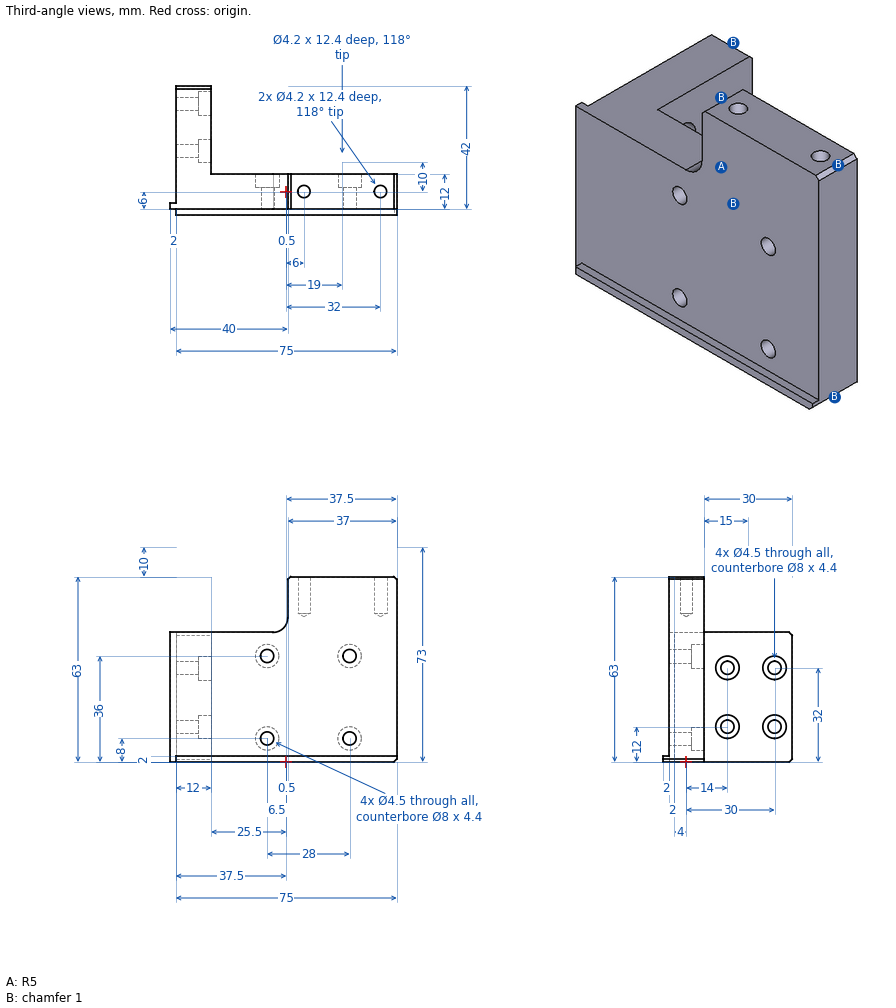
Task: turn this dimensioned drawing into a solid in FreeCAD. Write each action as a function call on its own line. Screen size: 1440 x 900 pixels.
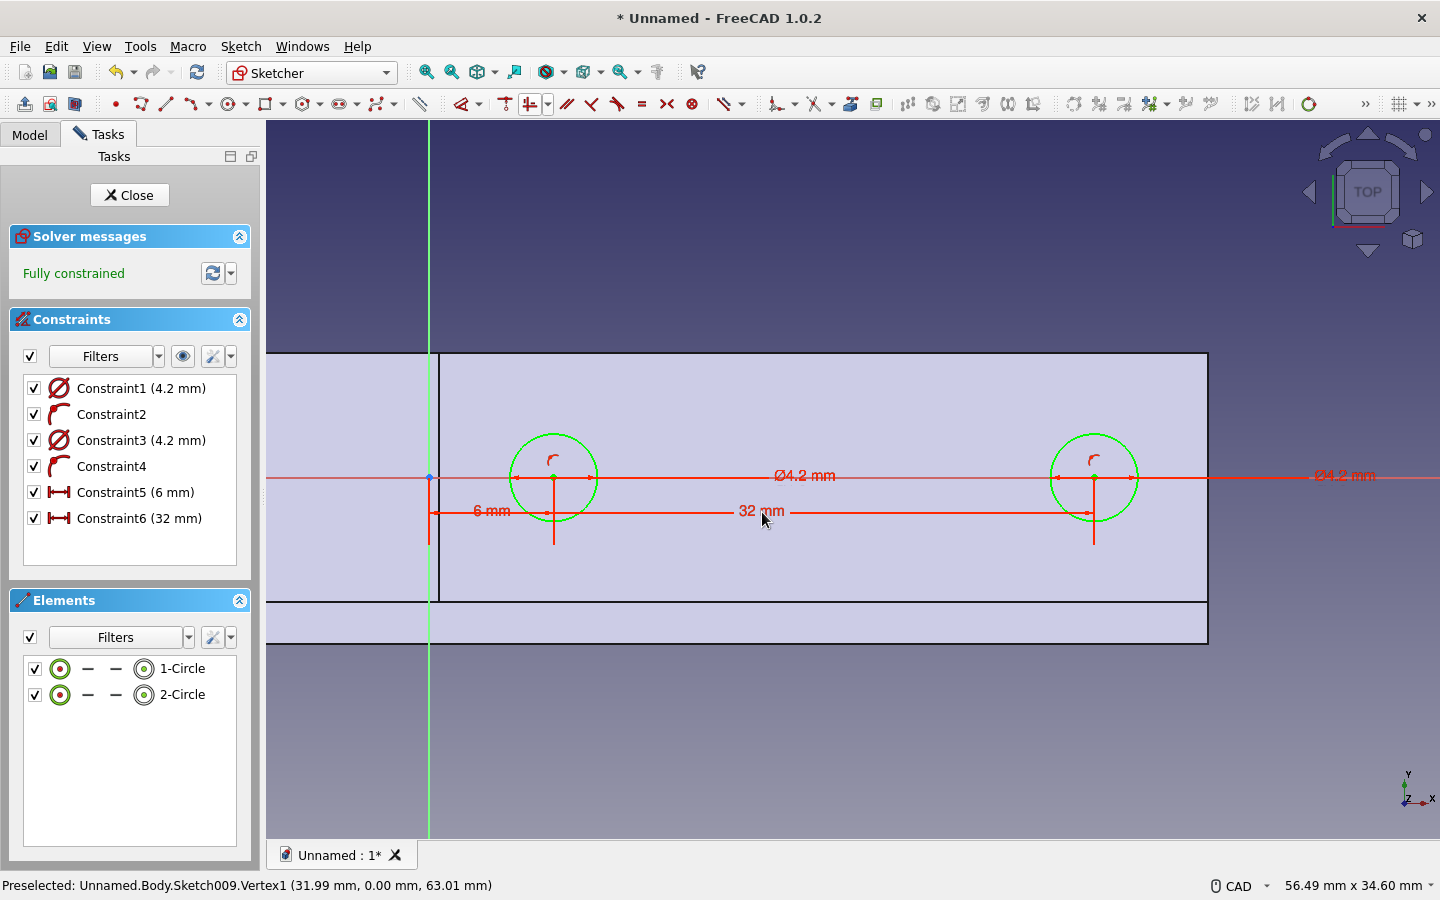
click(130, 195)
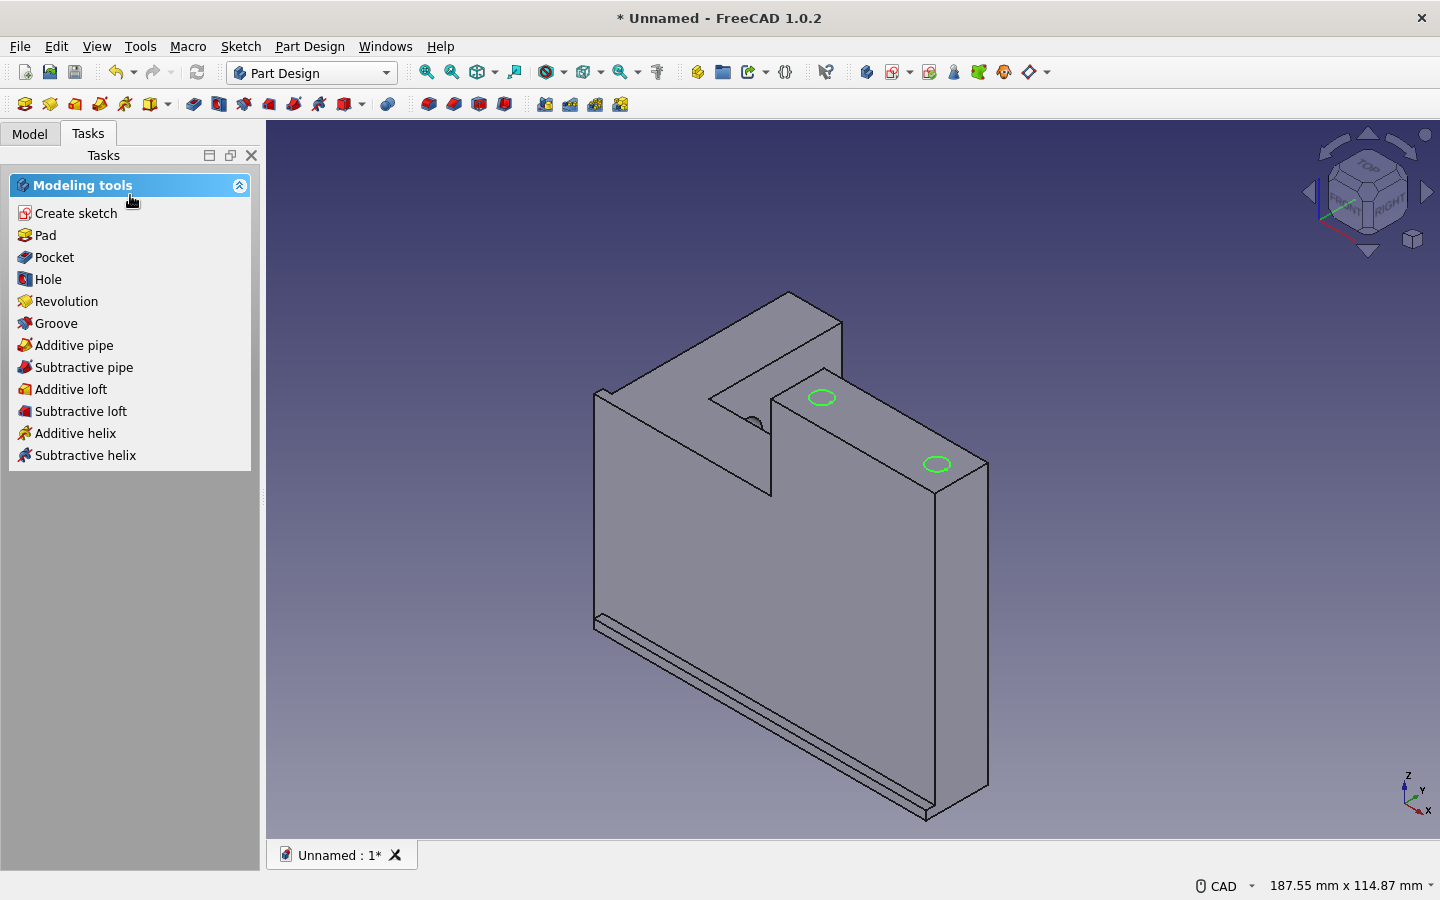
click(219, 104)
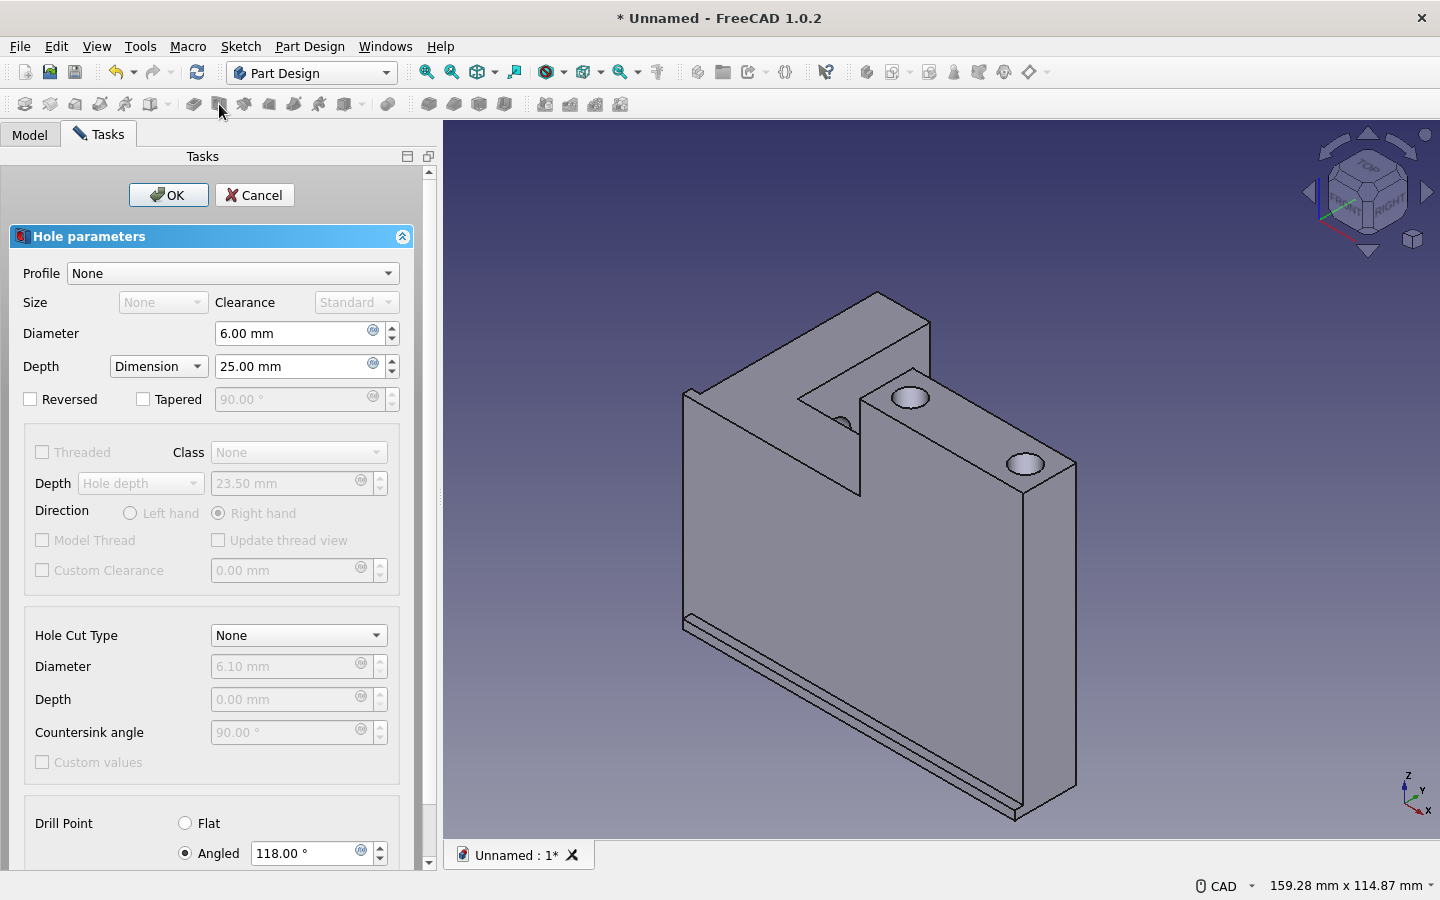
triple_click(300, 334)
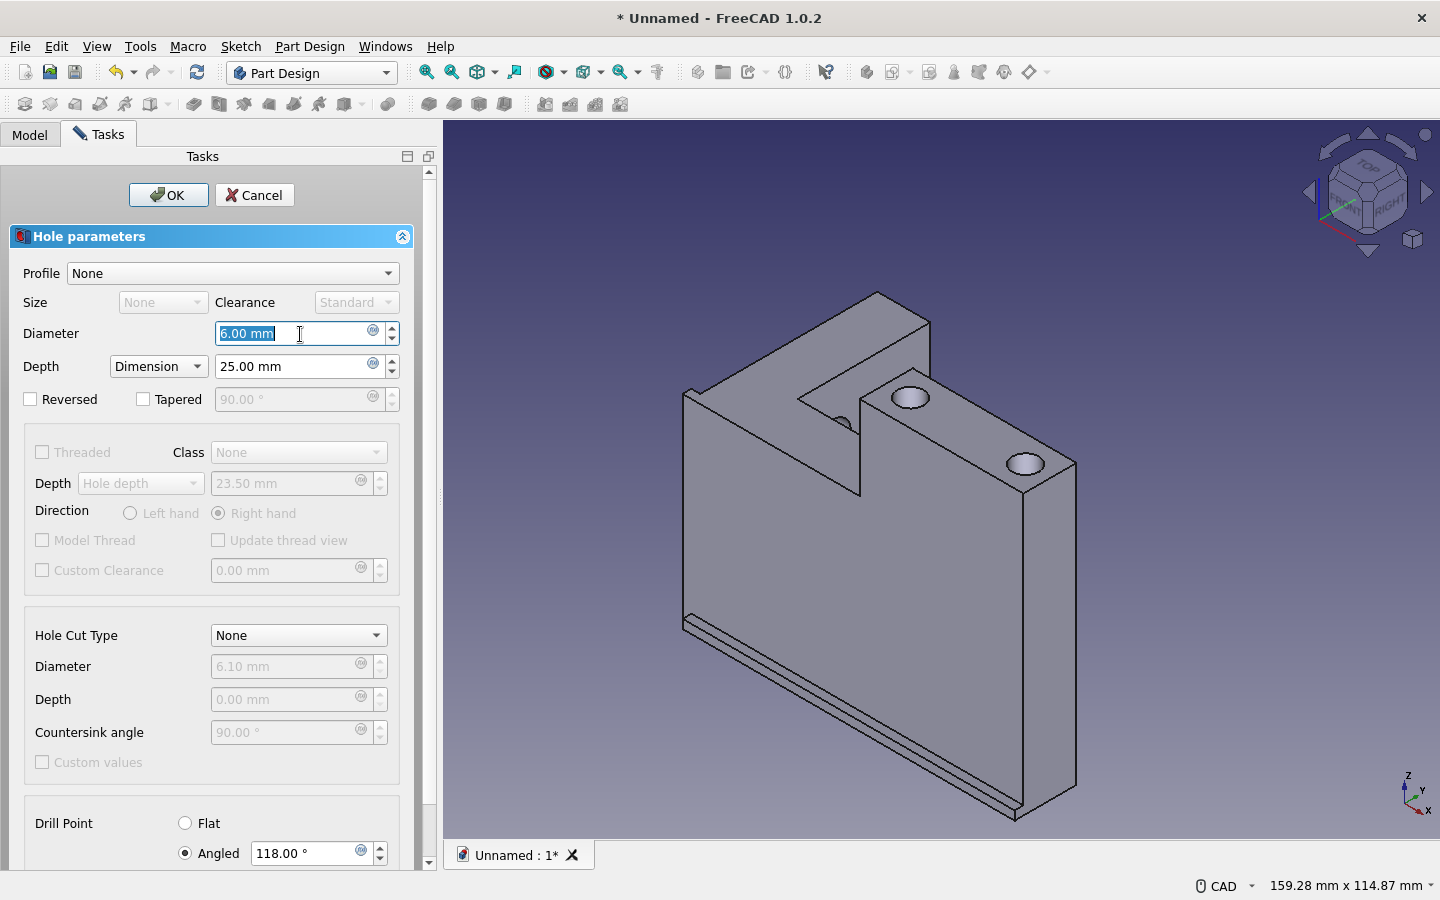
text(4.2)
key(Tab)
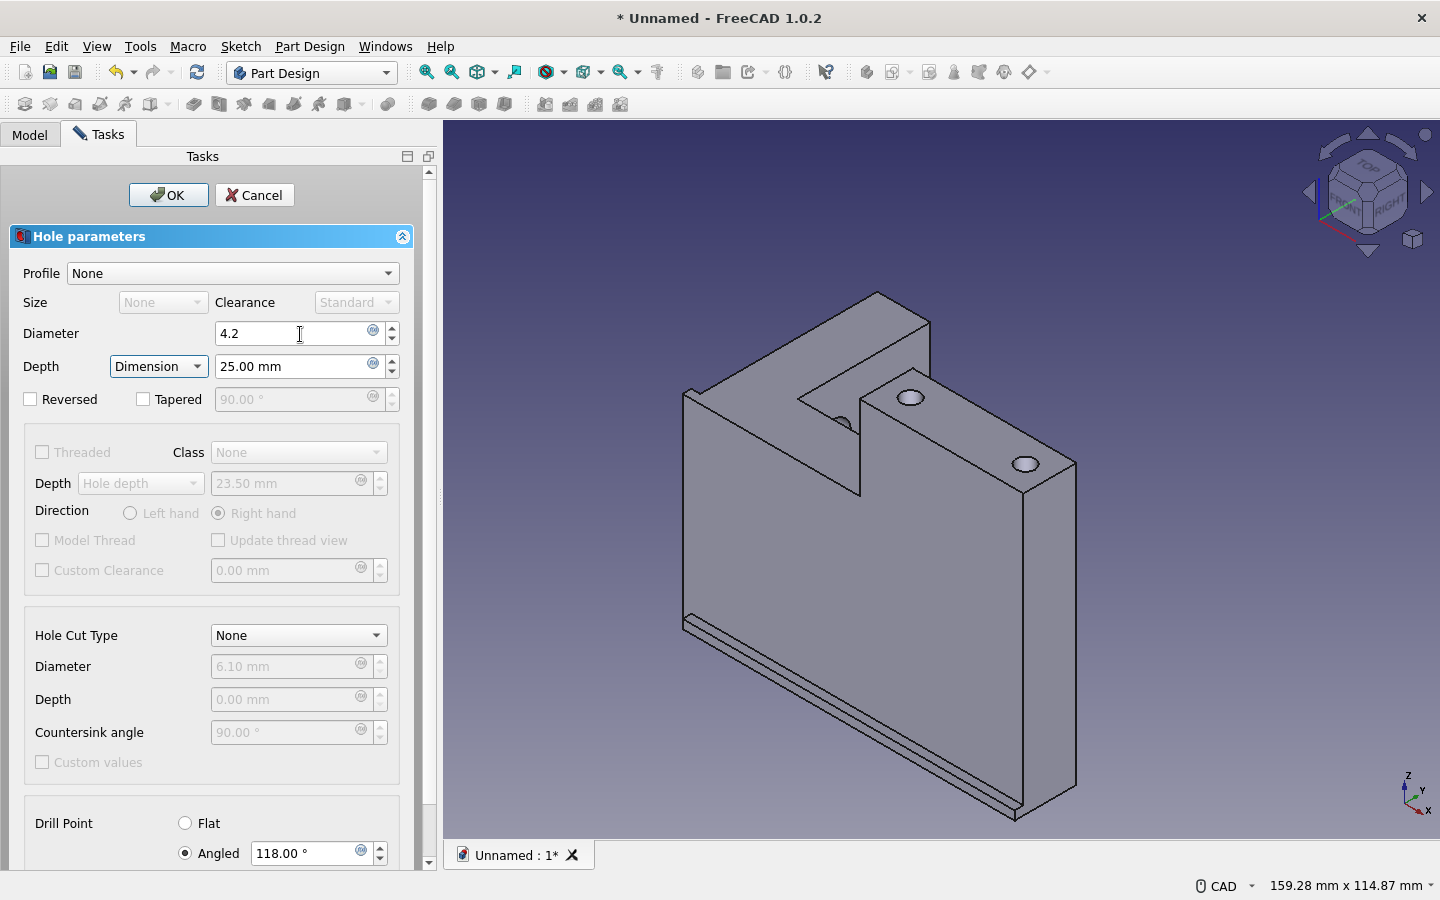
triple_click(300, 366)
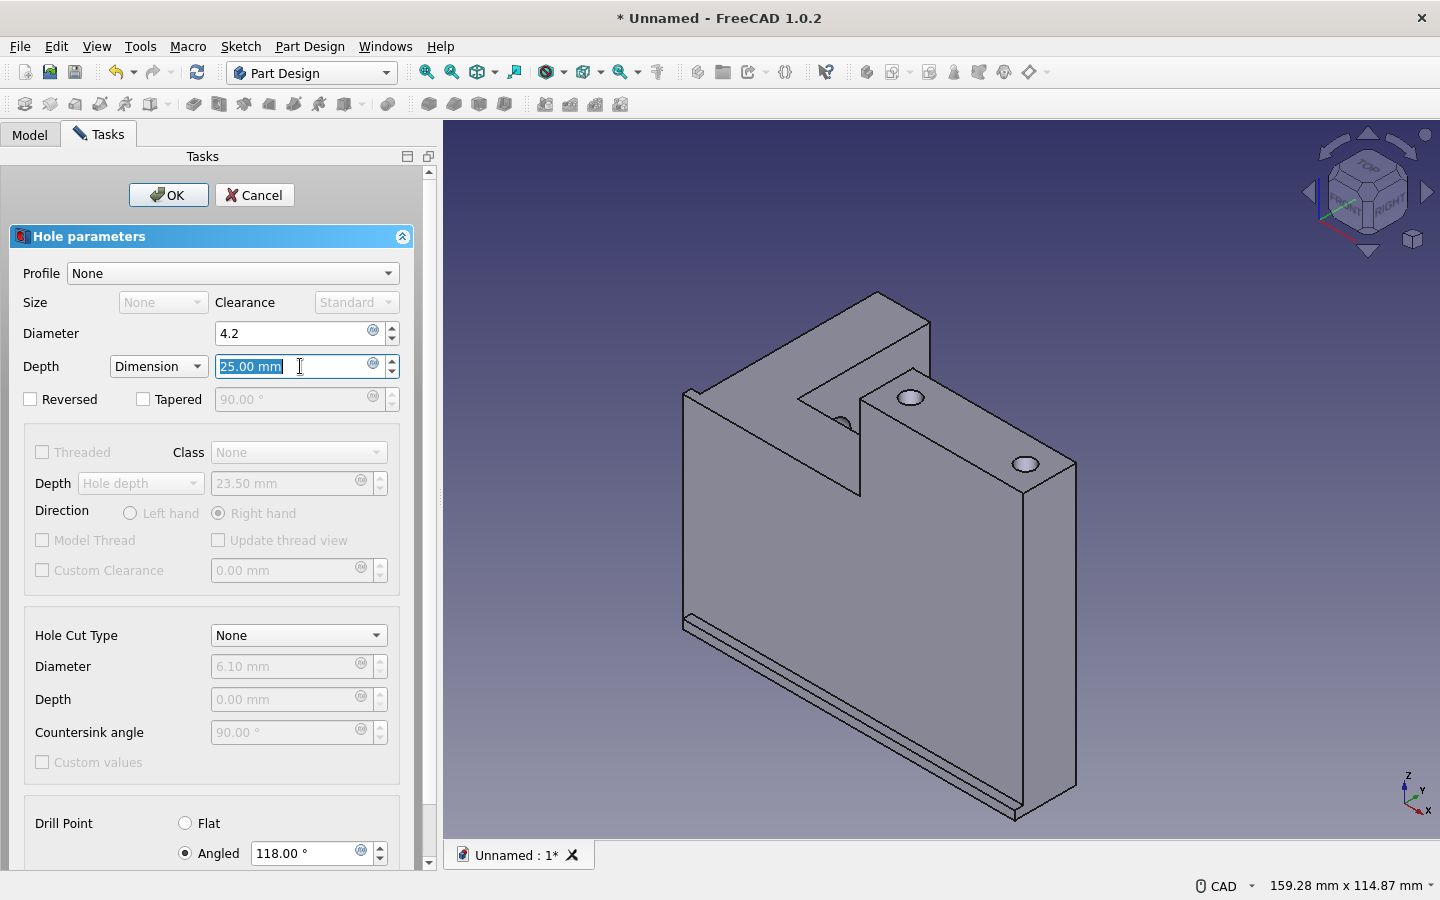
text(12.4)
key(Tab)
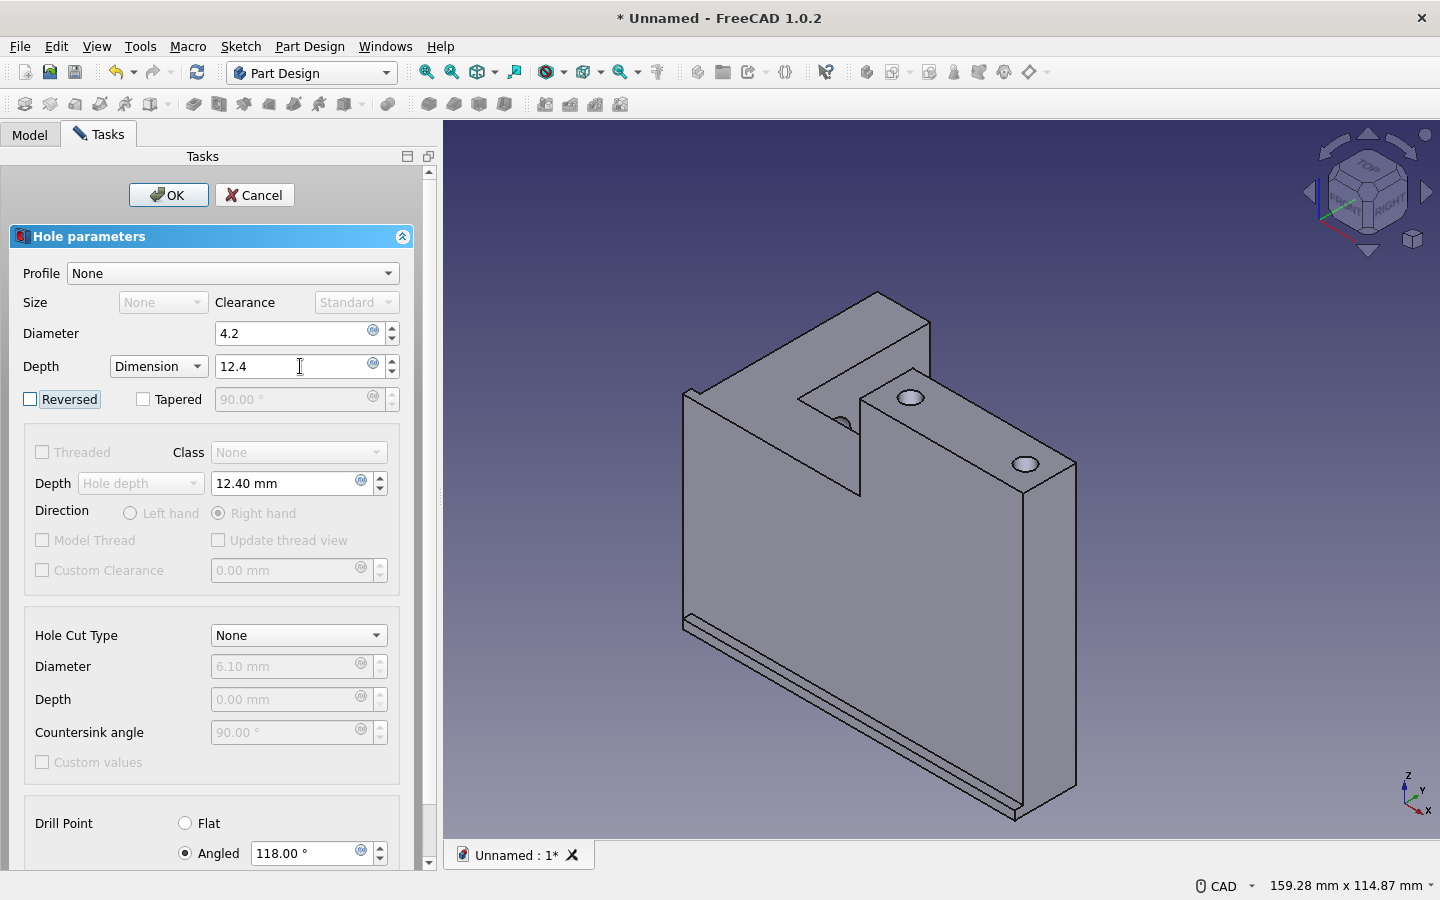
click(169, 195)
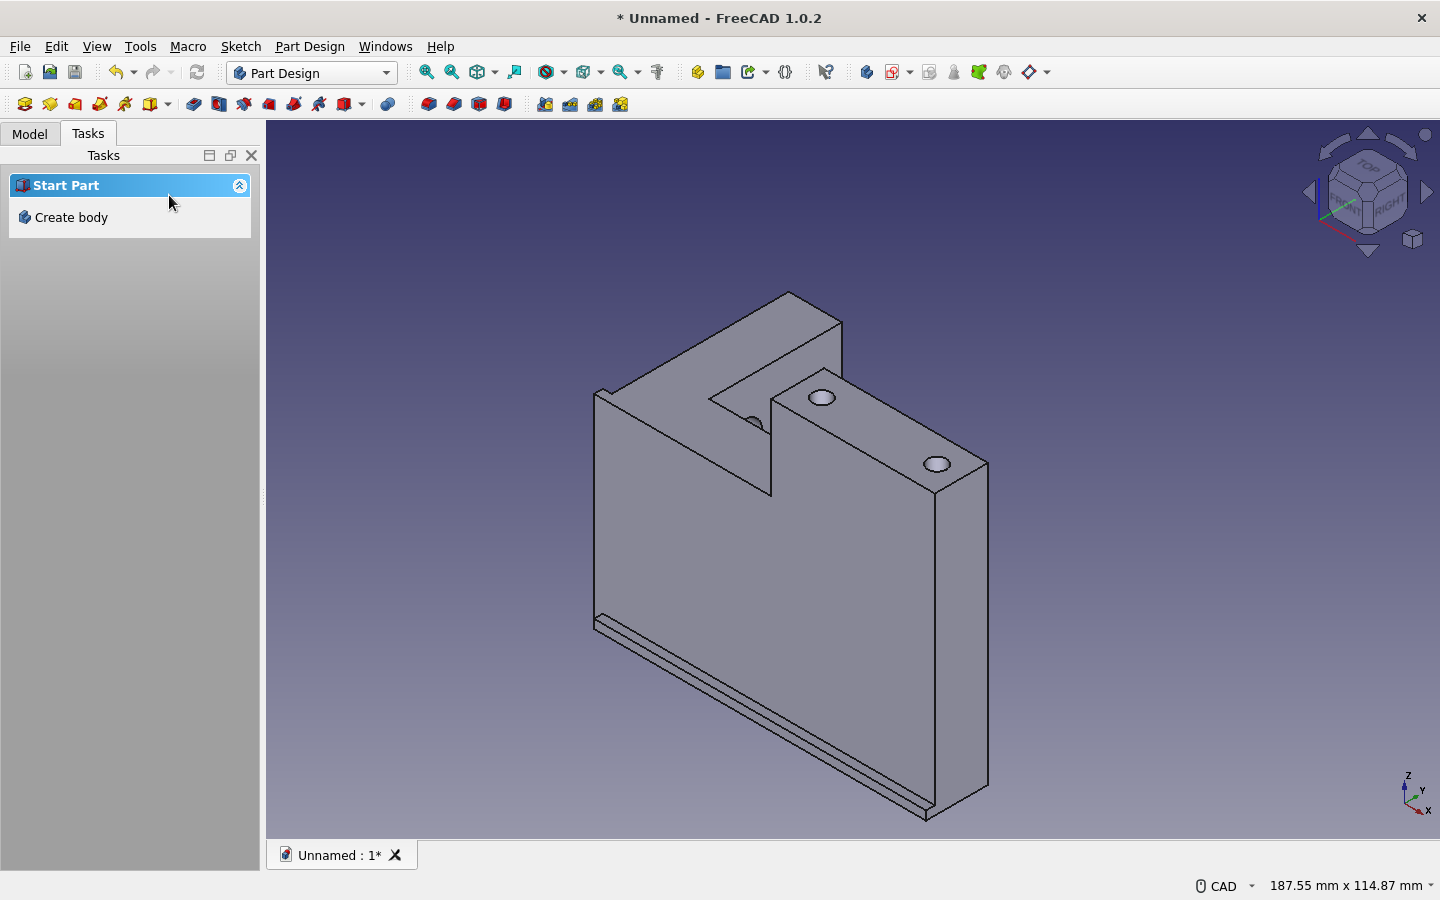
key(2)